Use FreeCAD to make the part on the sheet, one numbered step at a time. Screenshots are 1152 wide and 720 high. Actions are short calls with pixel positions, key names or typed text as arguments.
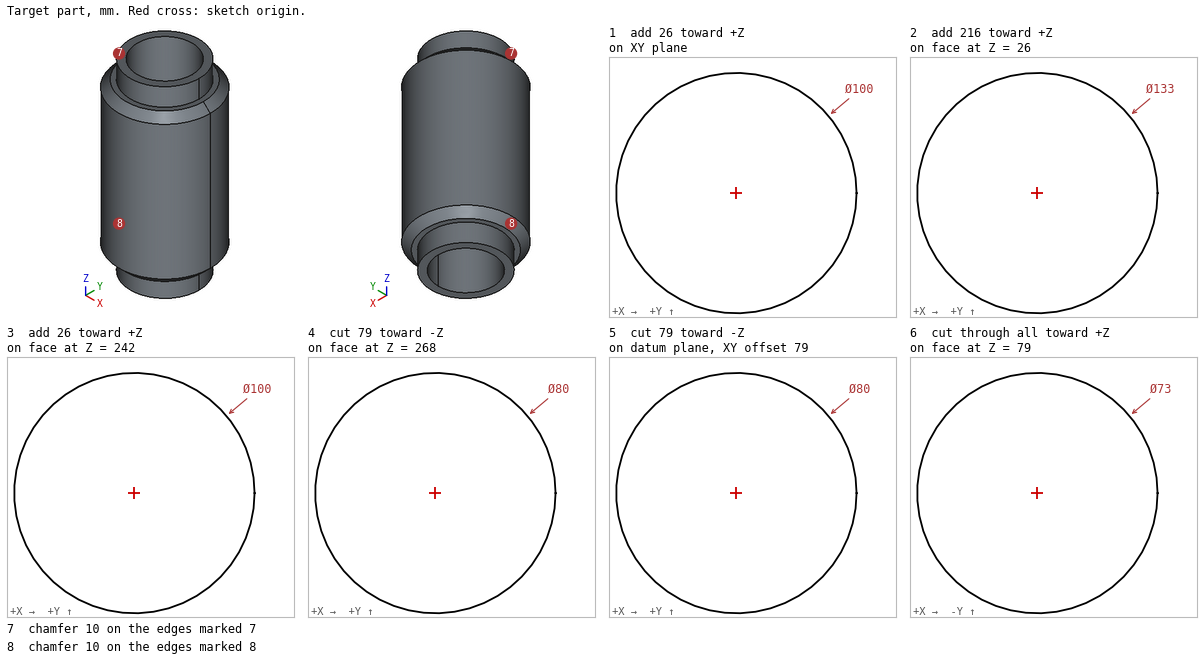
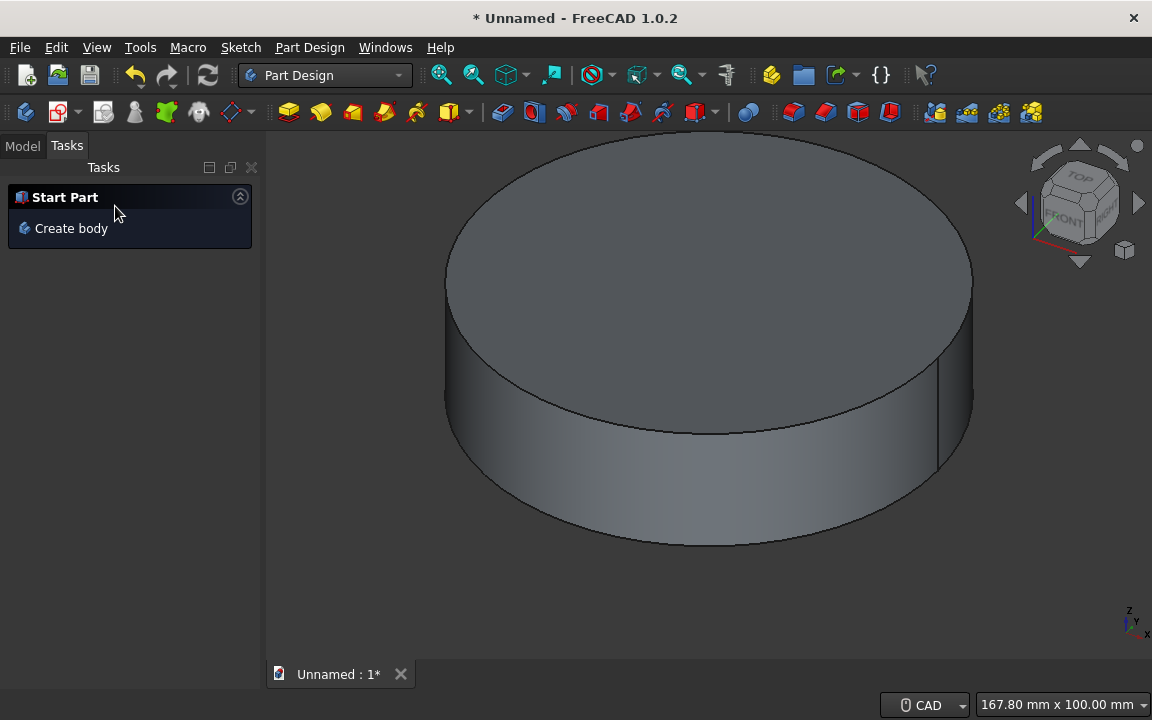
key(v)
key(f)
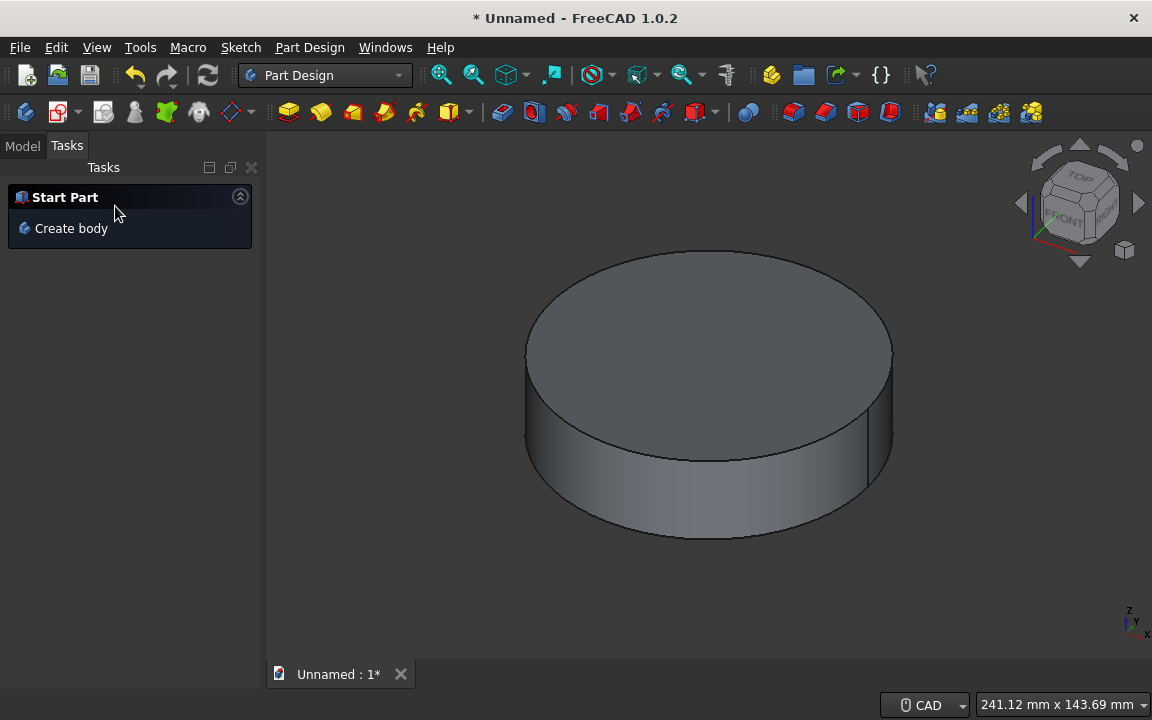
click(709, 355)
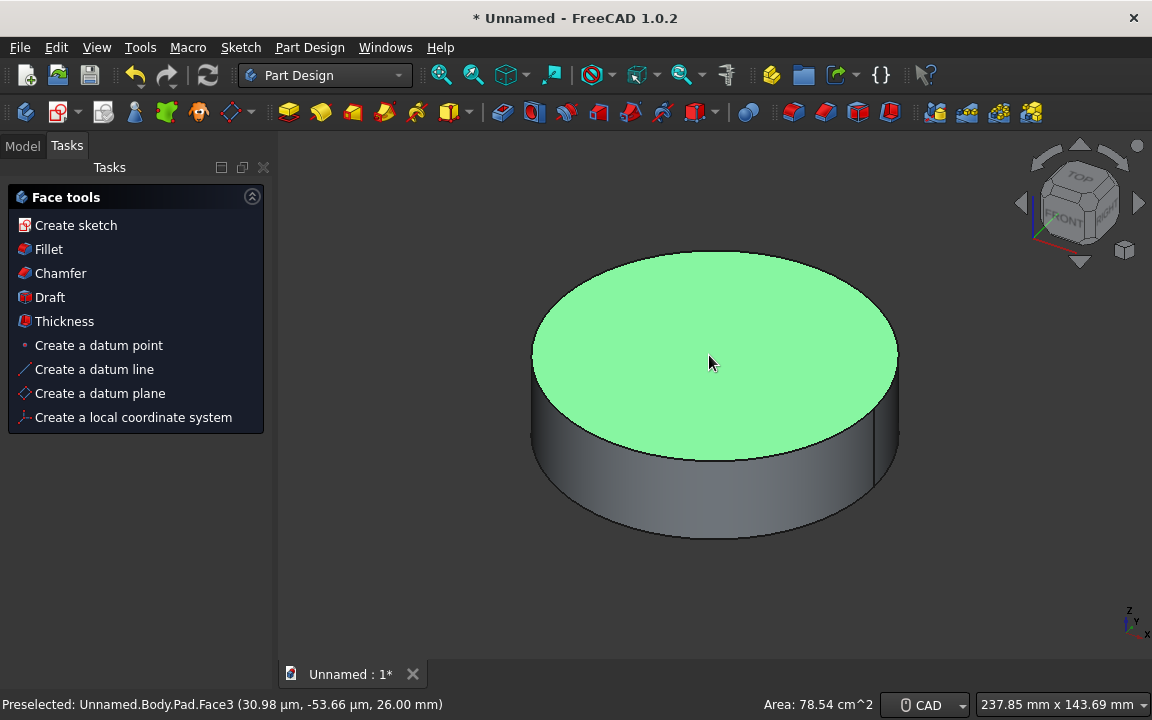
click(58, 112)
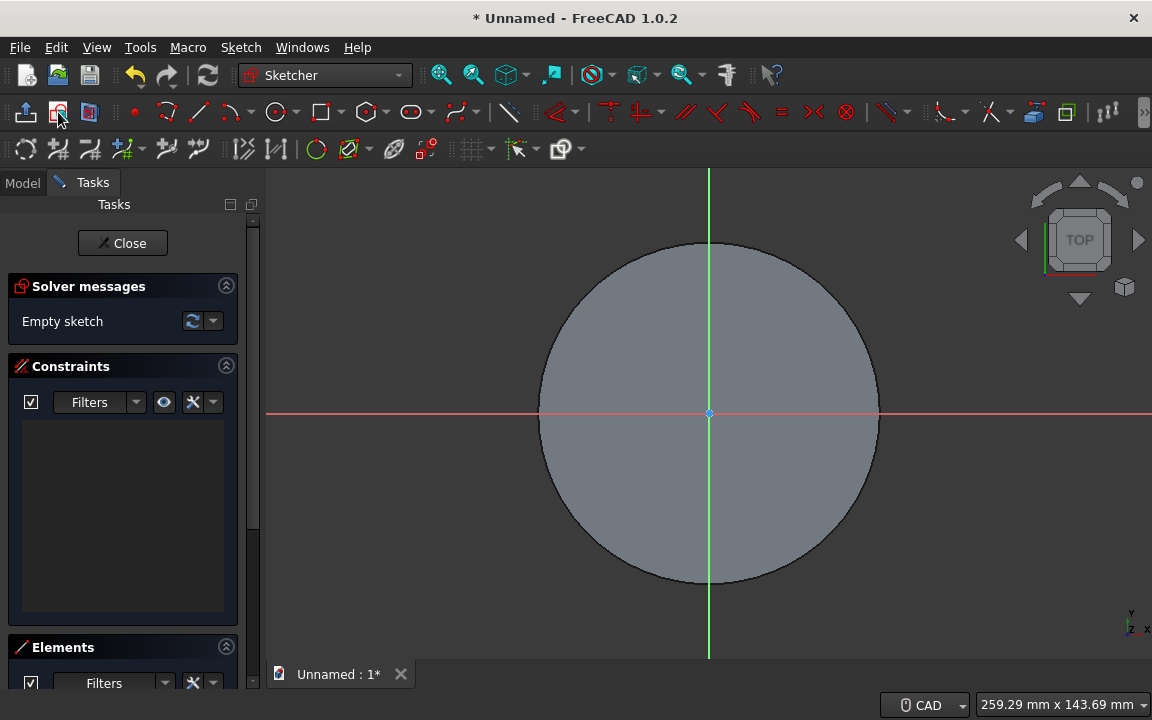
scroll(501, 414, down, 2)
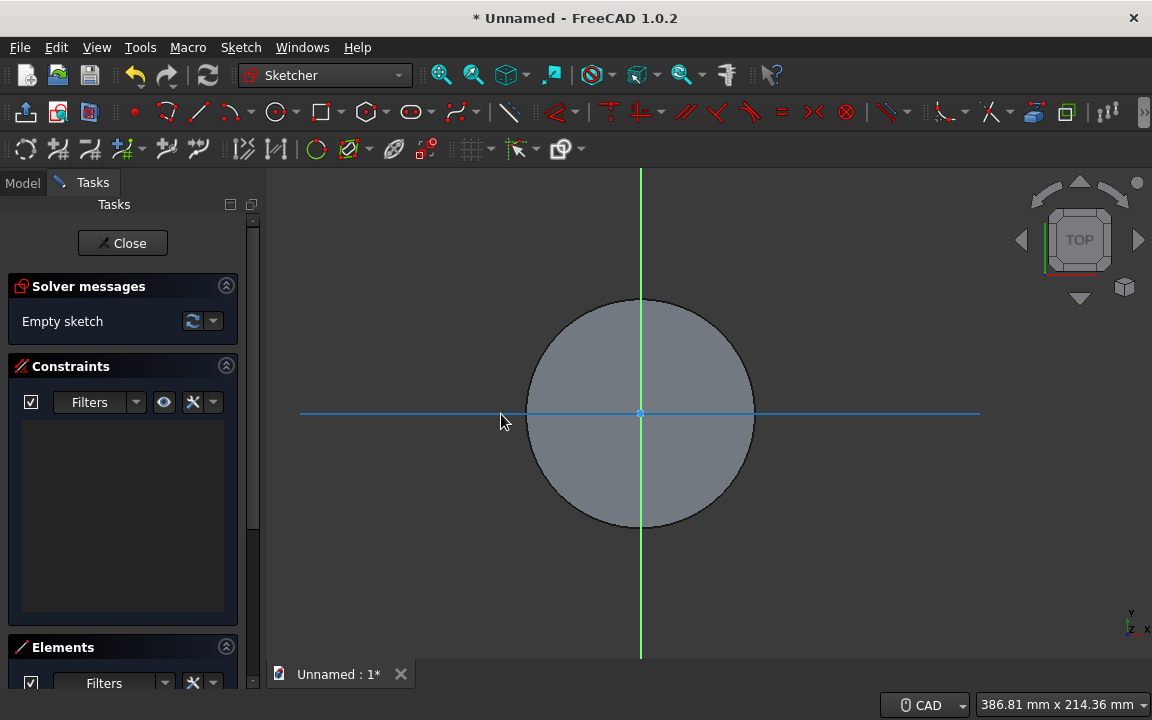
click(276, 112)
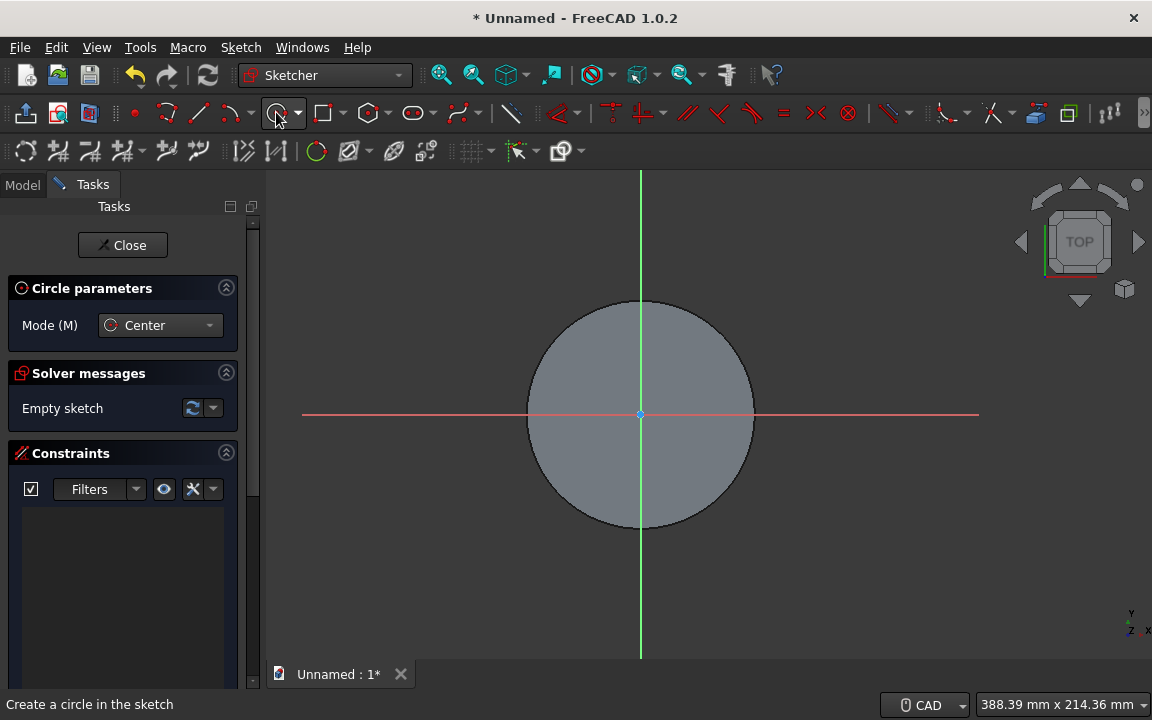
click(641, 415)
move(748, 308)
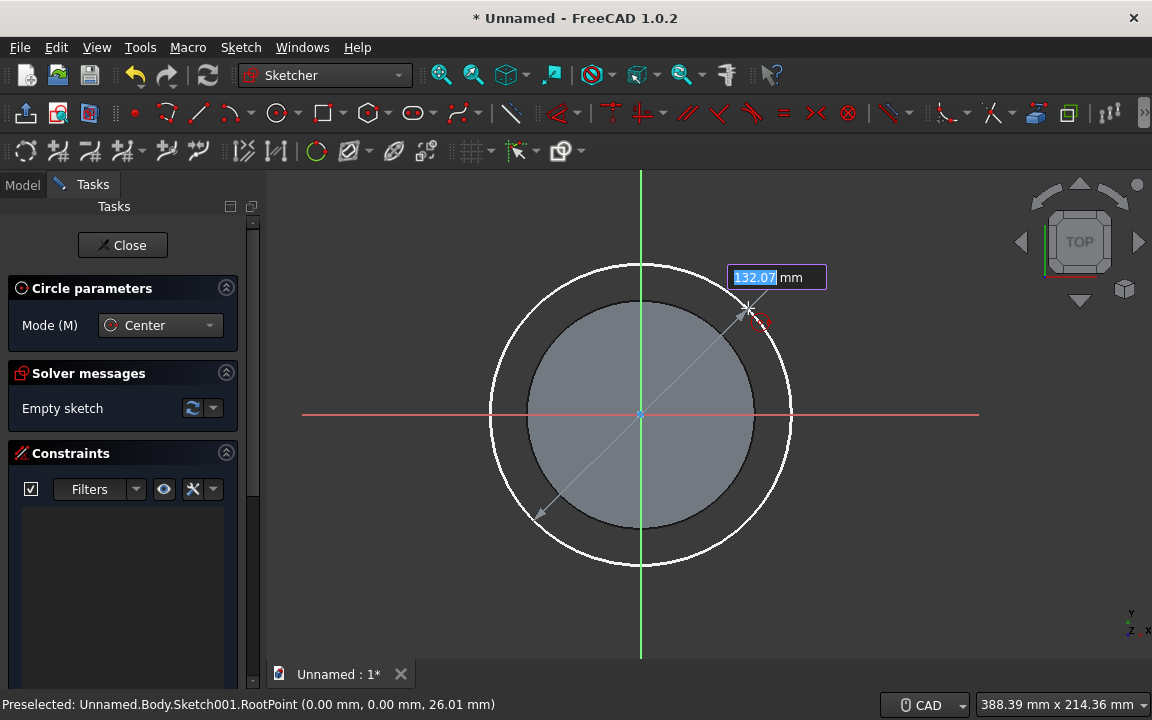
text(133)
key(Return)
key(Escape)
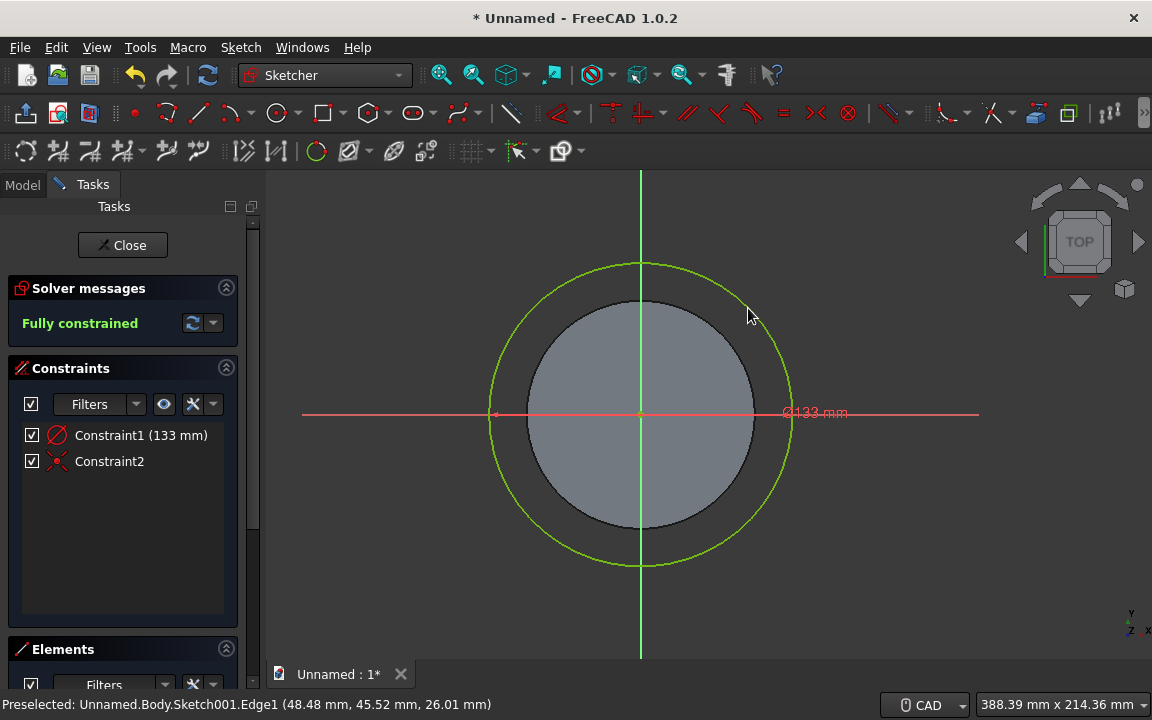
click(123, 245)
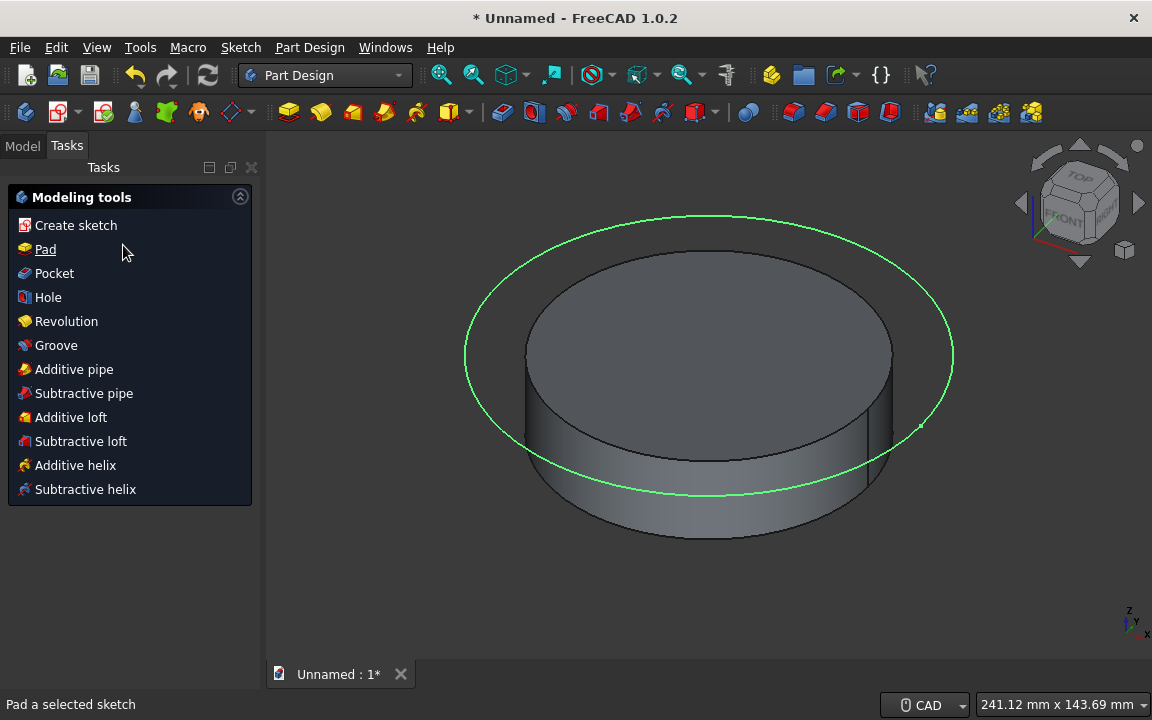
click(290, 112)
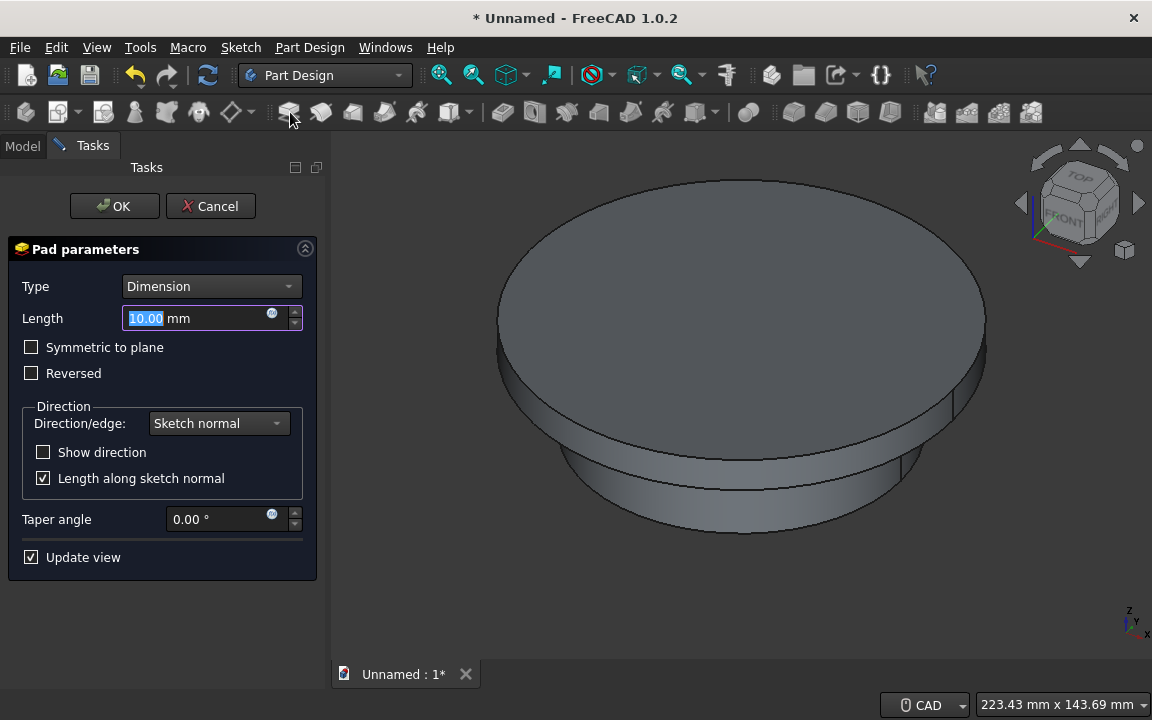
text(216)
key(Tab)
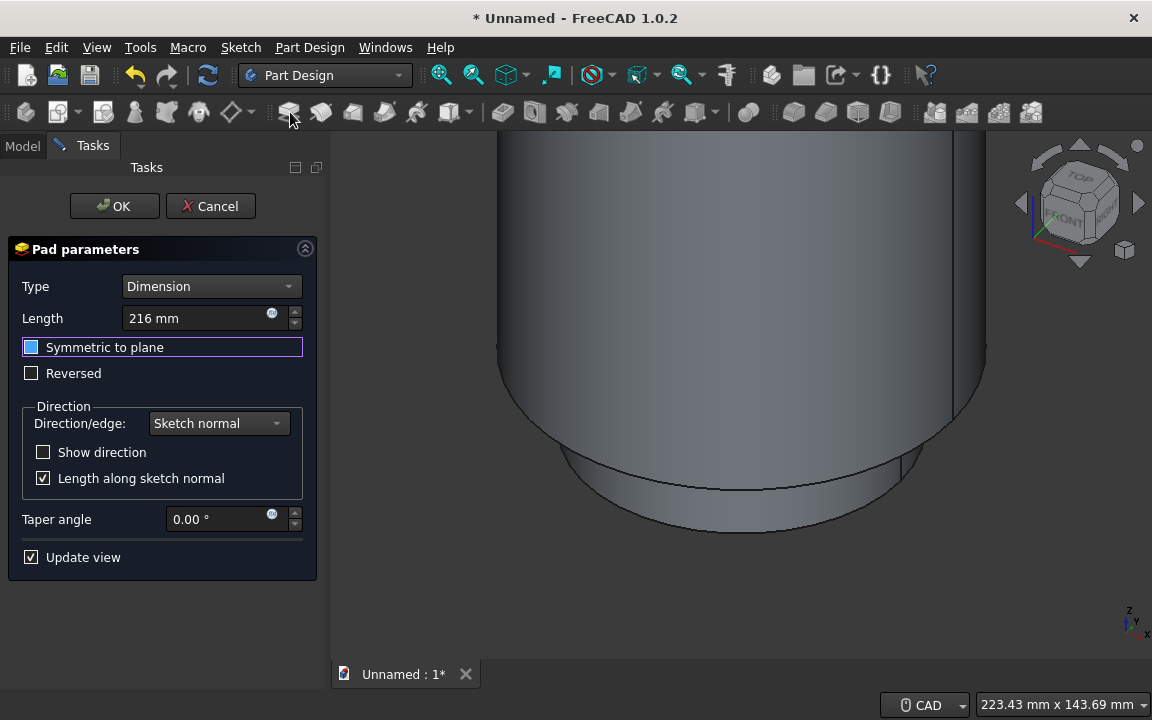
click(115, 206)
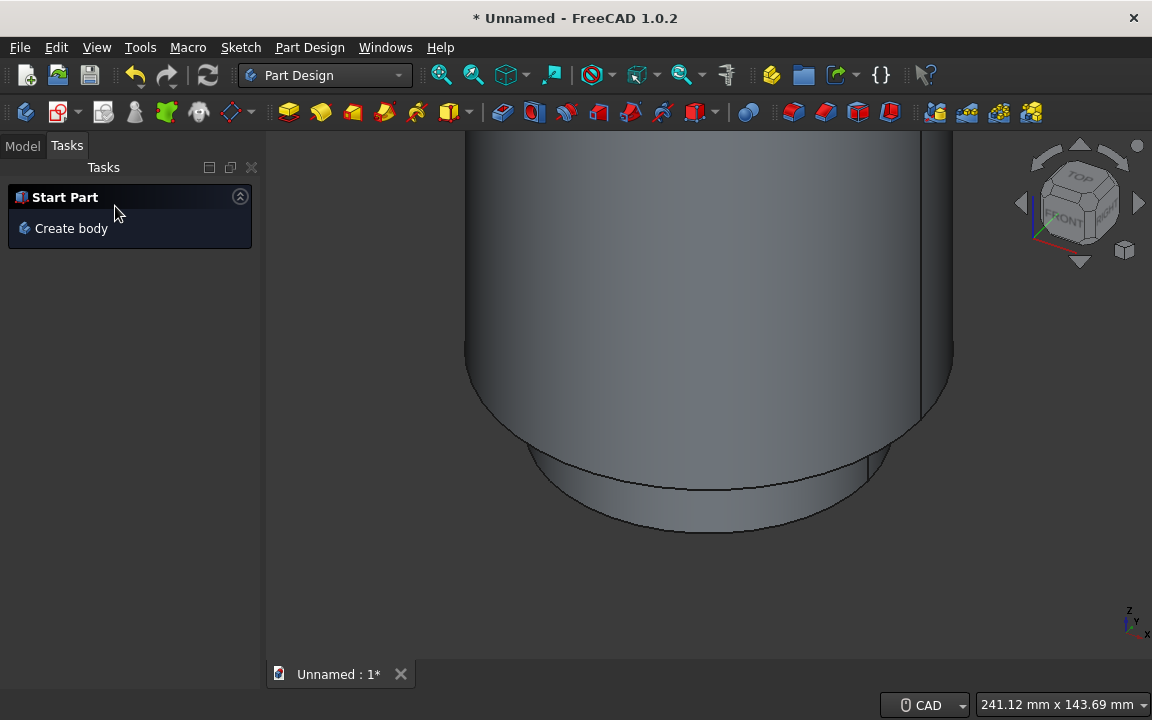
key(v)
key(f)